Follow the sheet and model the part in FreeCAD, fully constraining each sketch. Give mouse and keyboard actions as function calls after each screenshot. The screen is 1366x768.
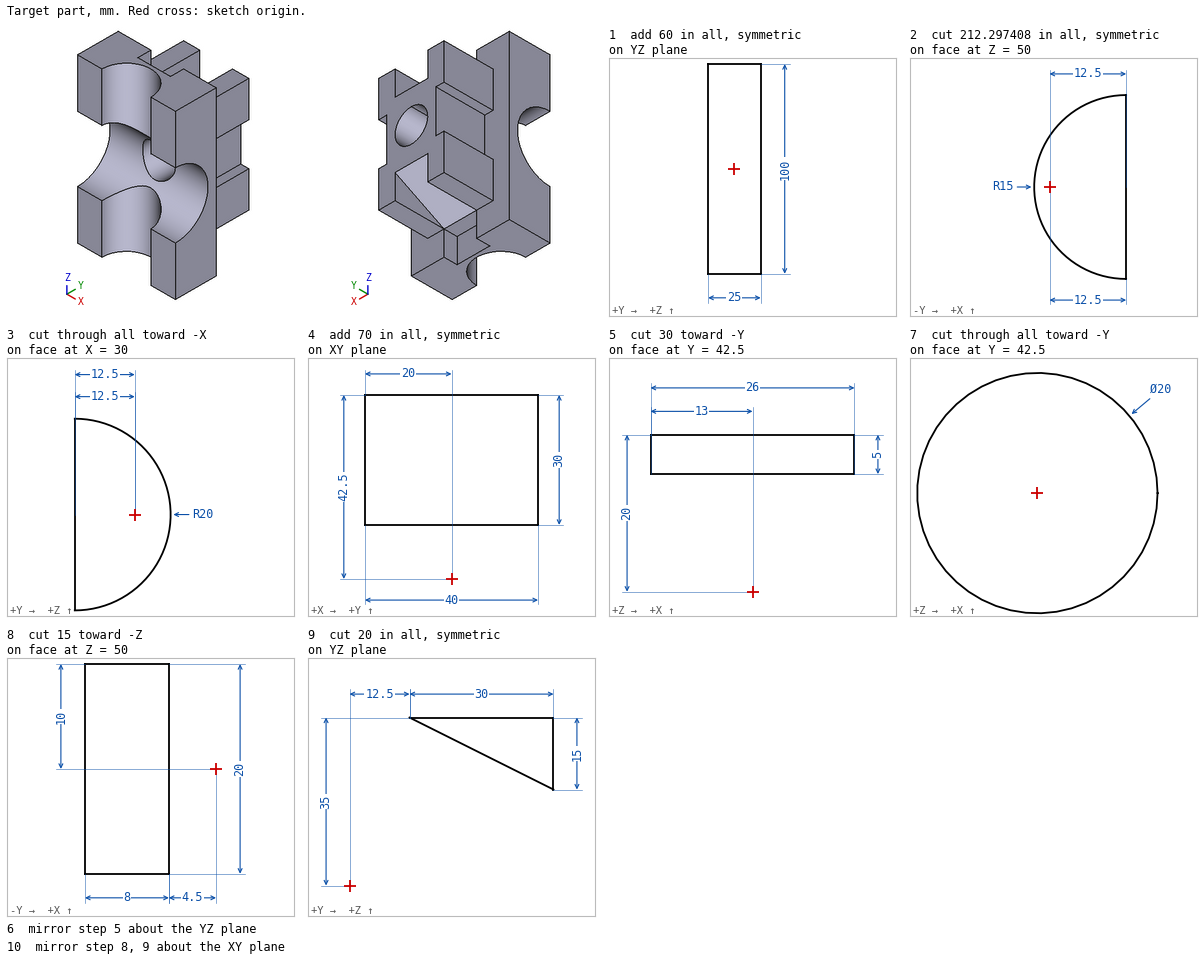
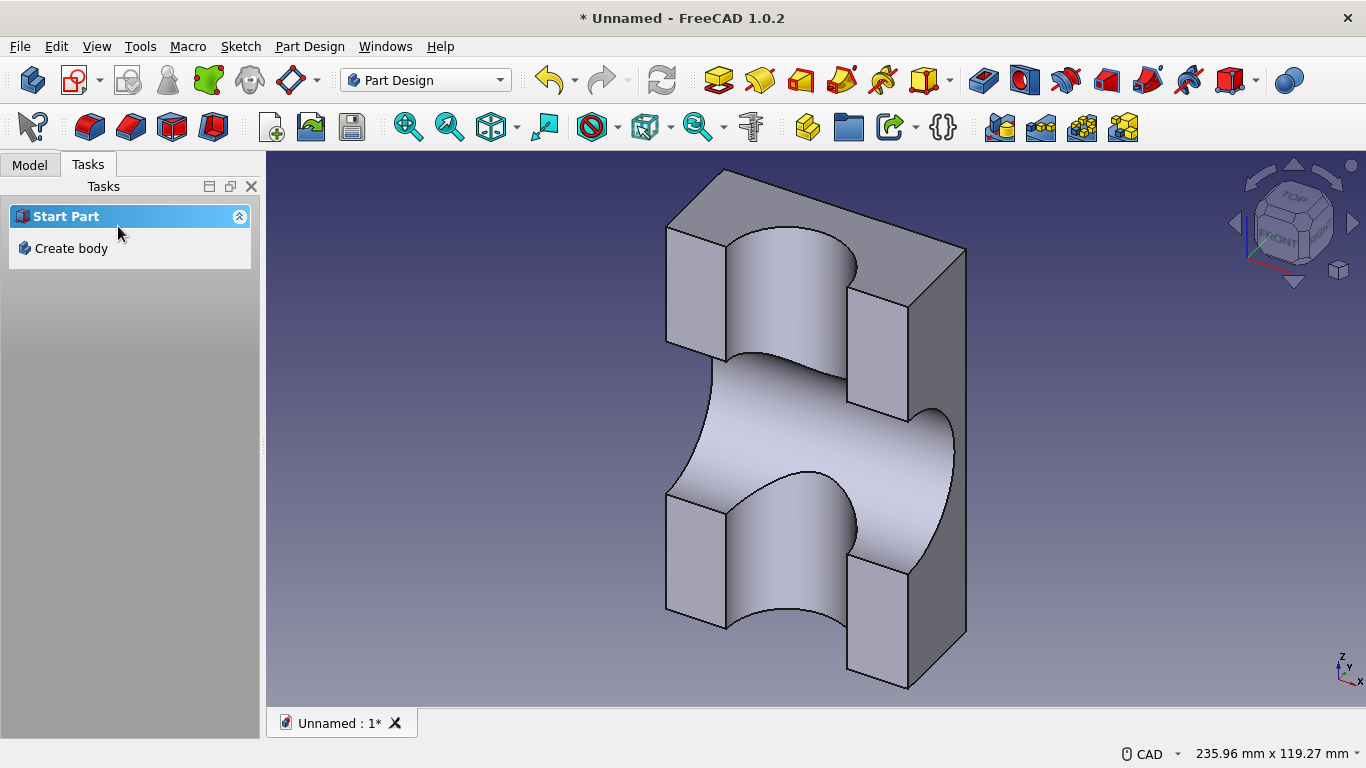
click(74, 80)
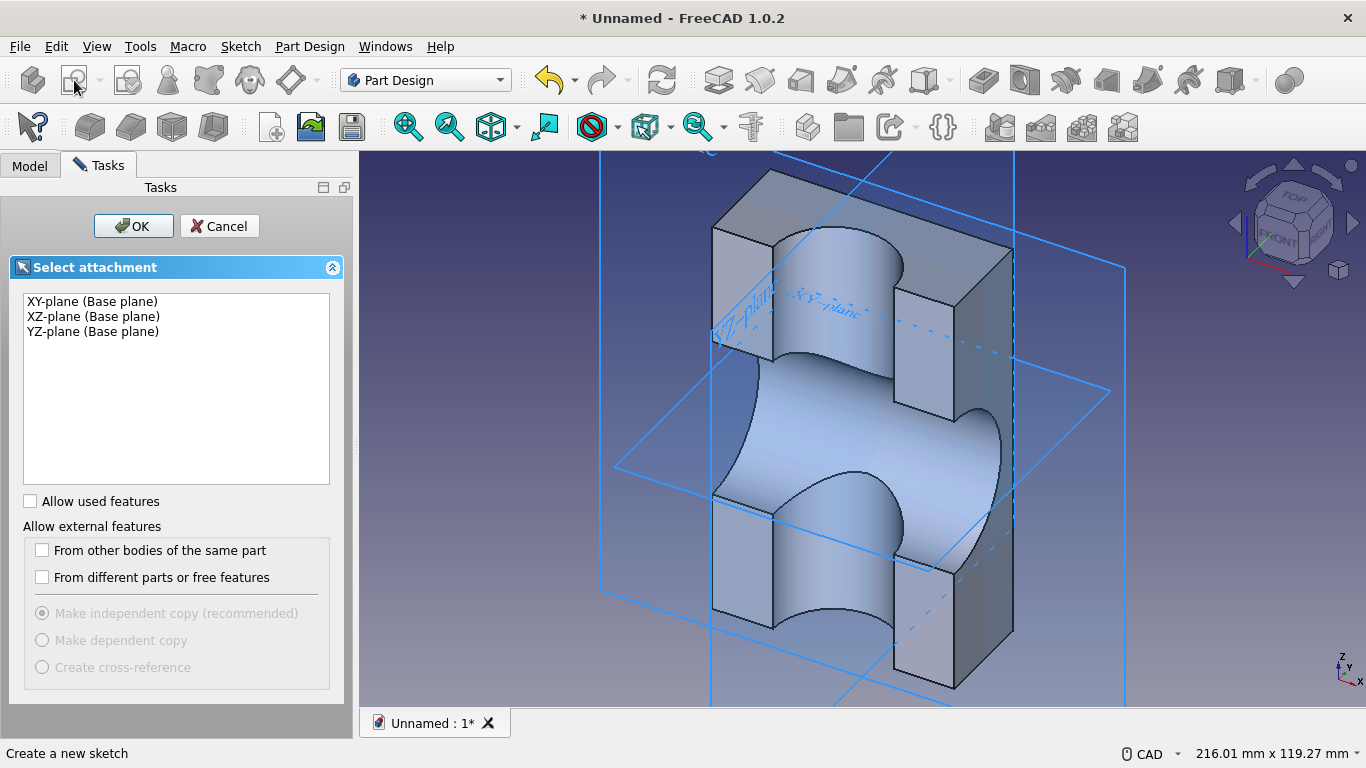
click(84, 302)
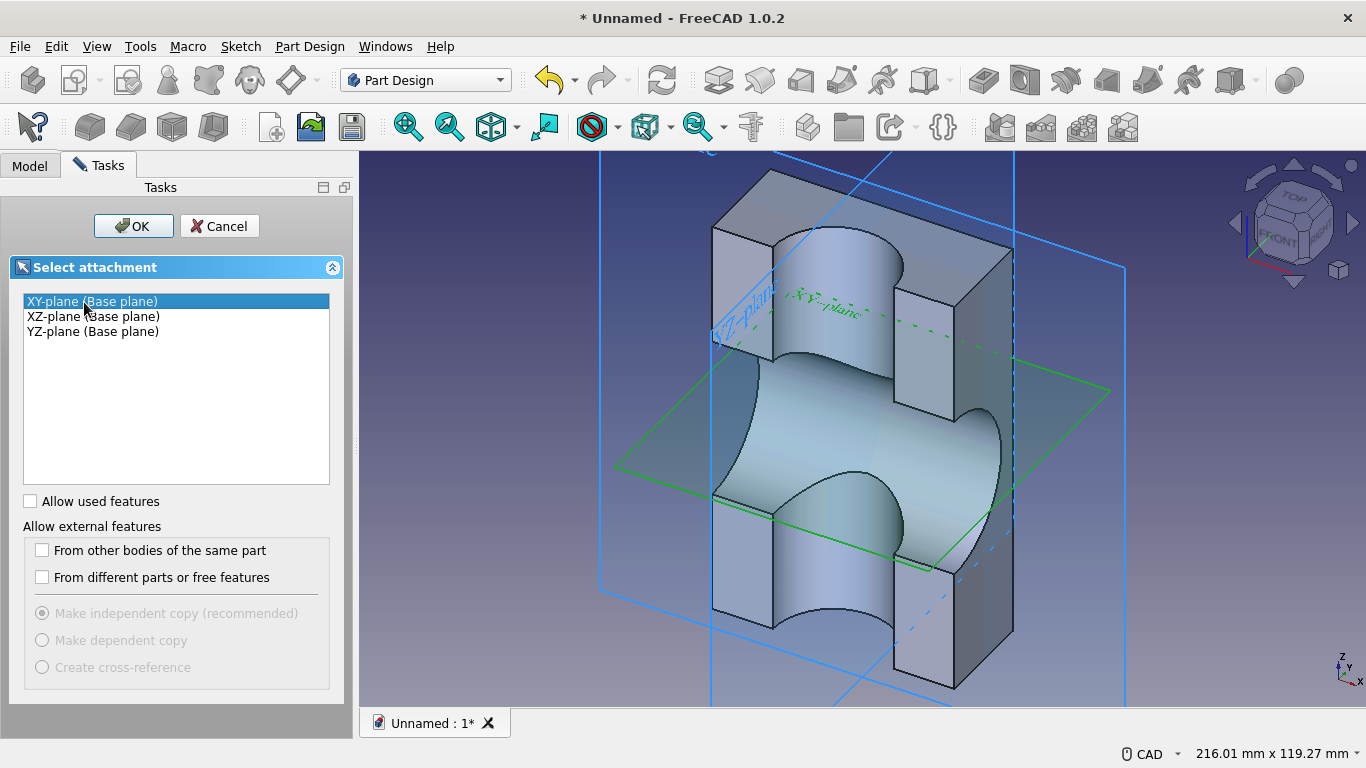
click(134, 226)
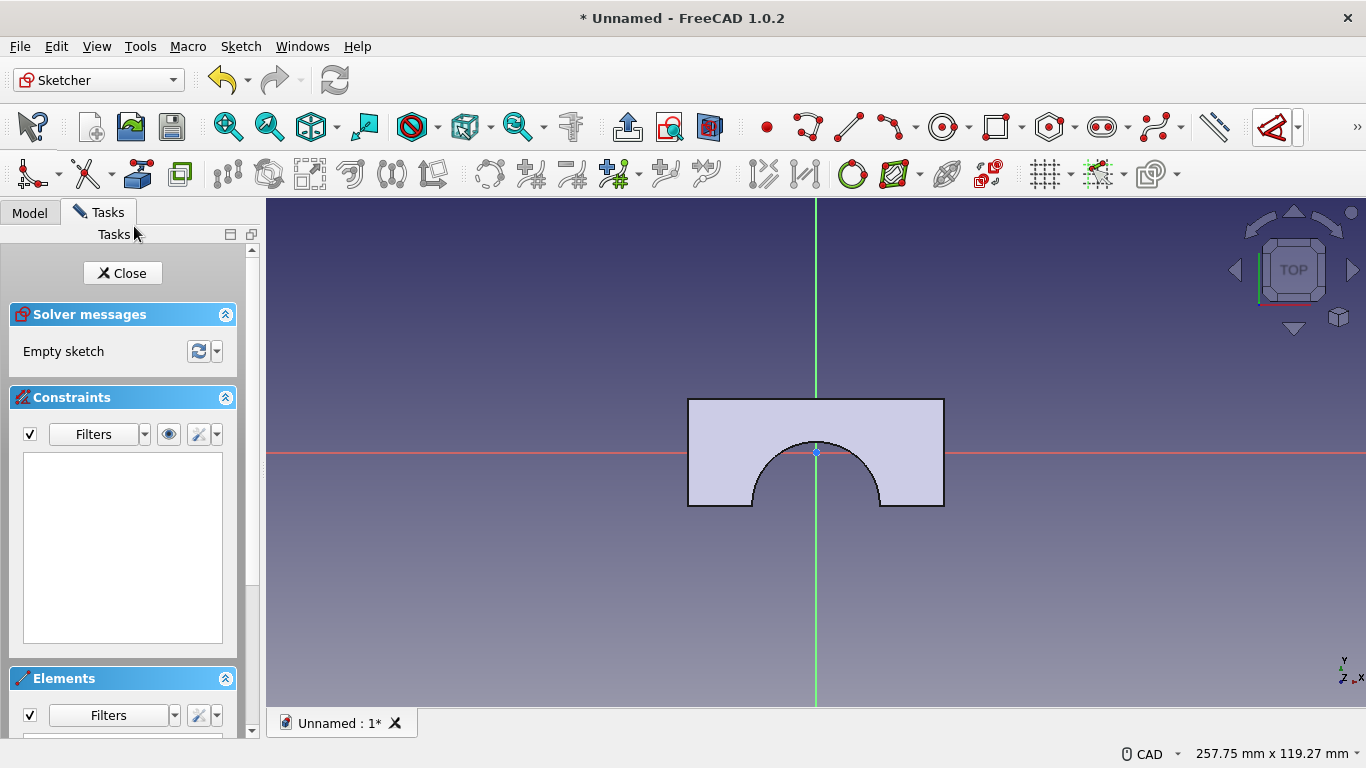
click(710, 128)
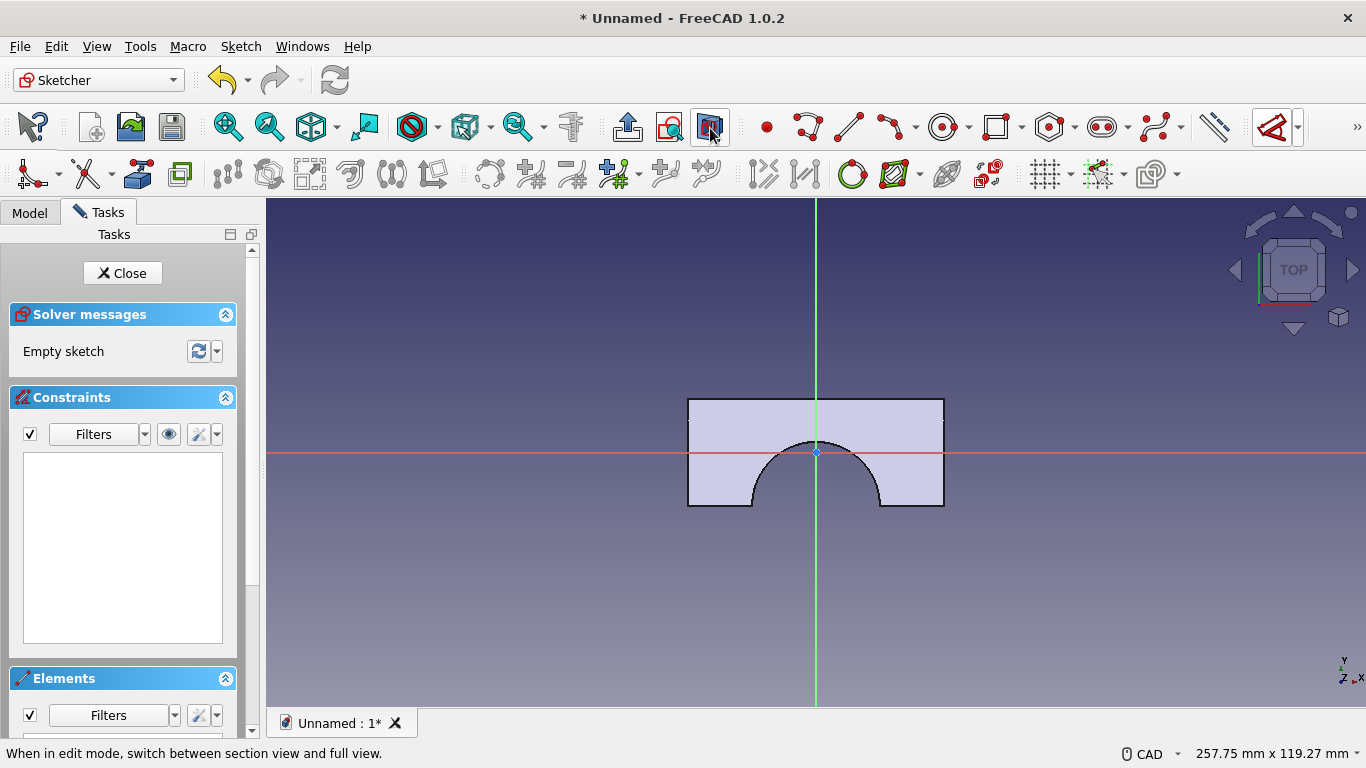
scroll(899, 252, up, 3)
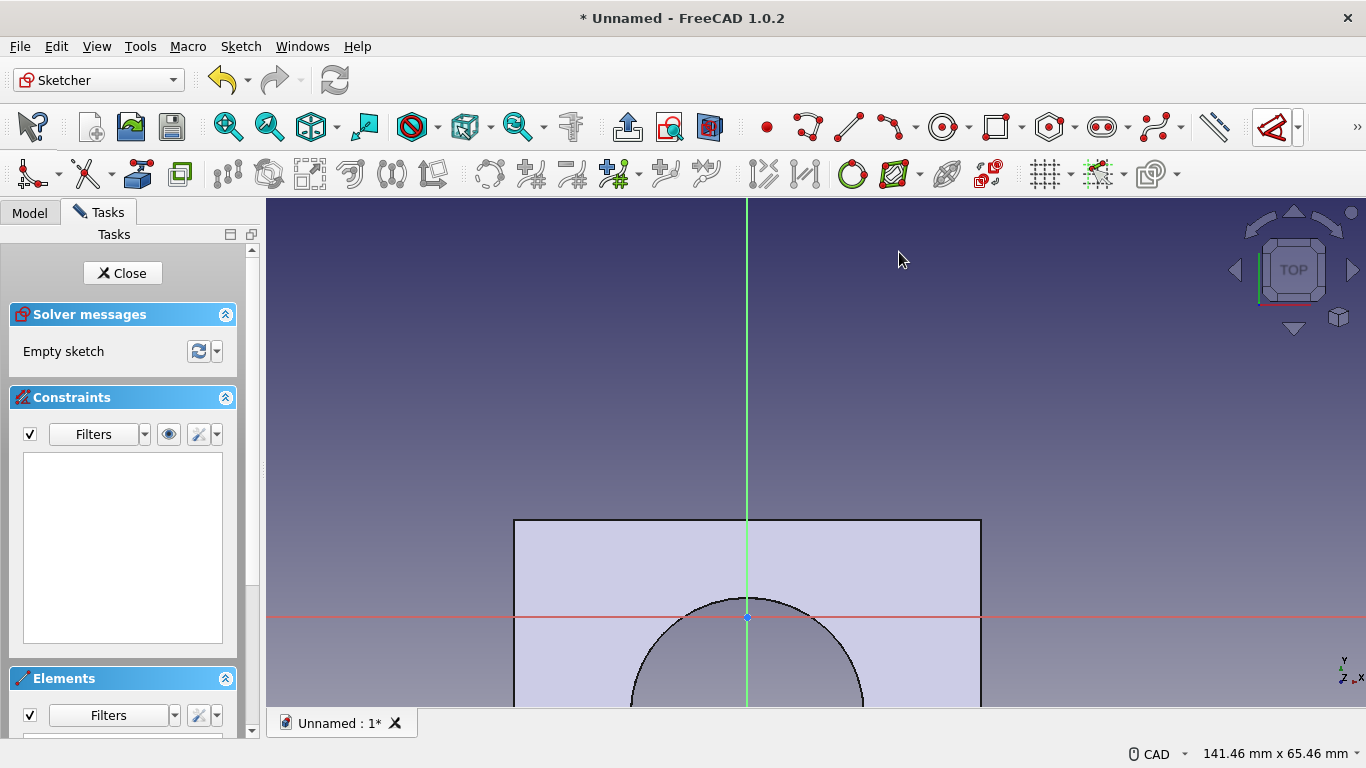
click(996, 128)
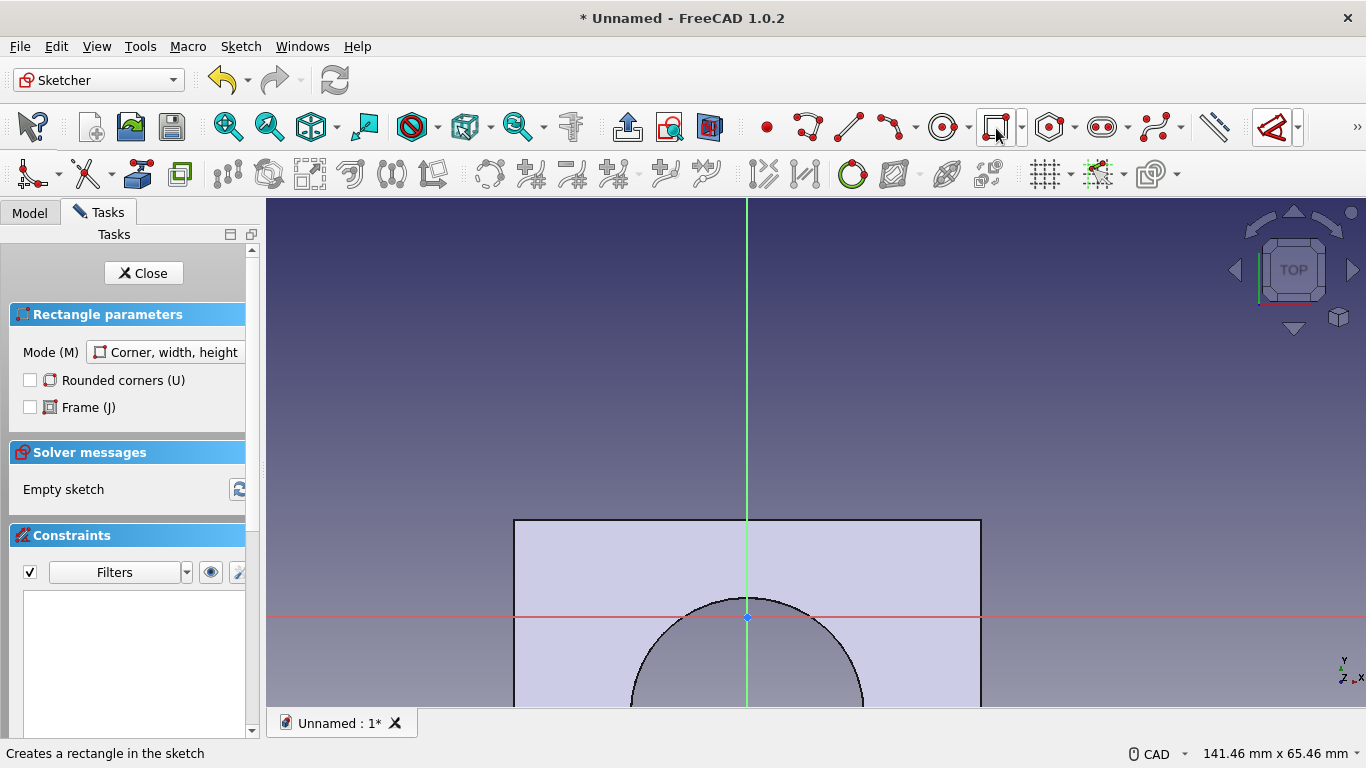
click(592, 287)
move(903, 520)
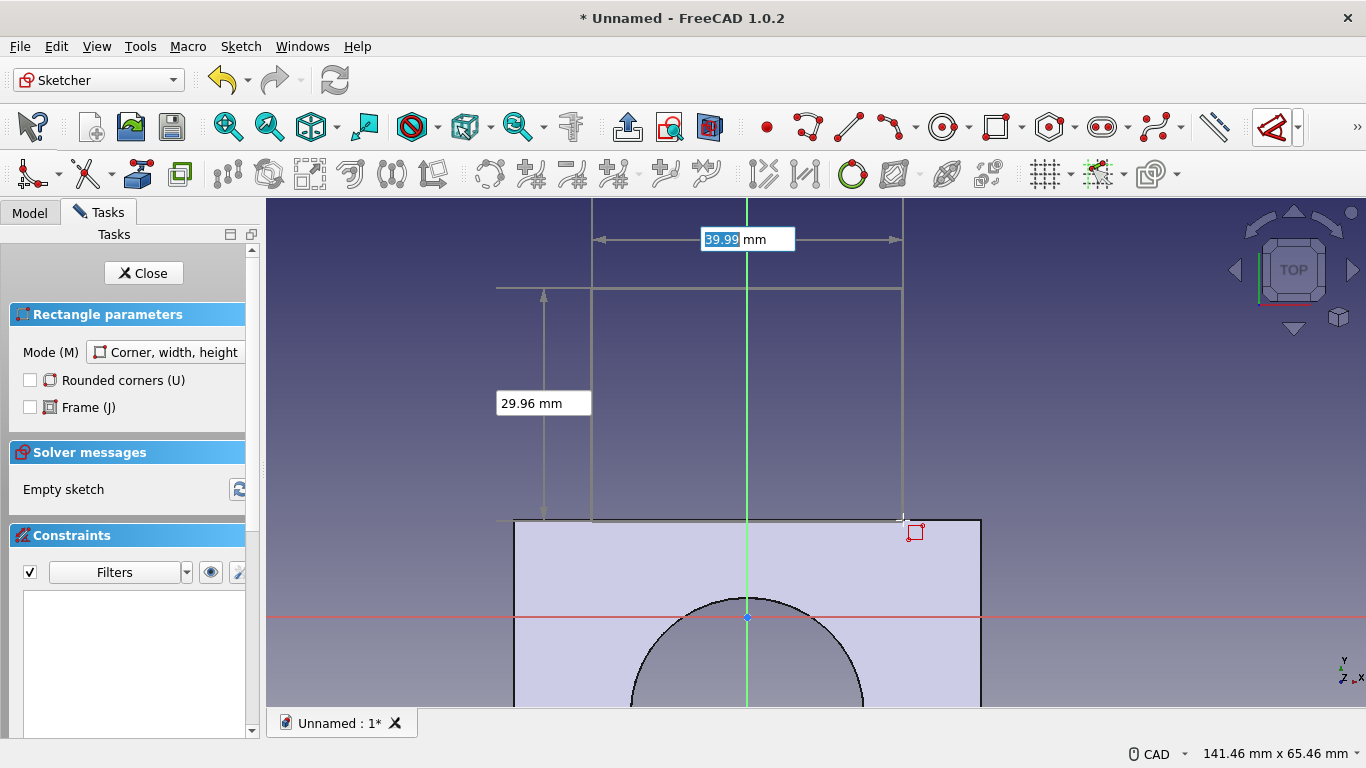
text(40)
key(Tab)
text(30)
key(Return)
key(Escape)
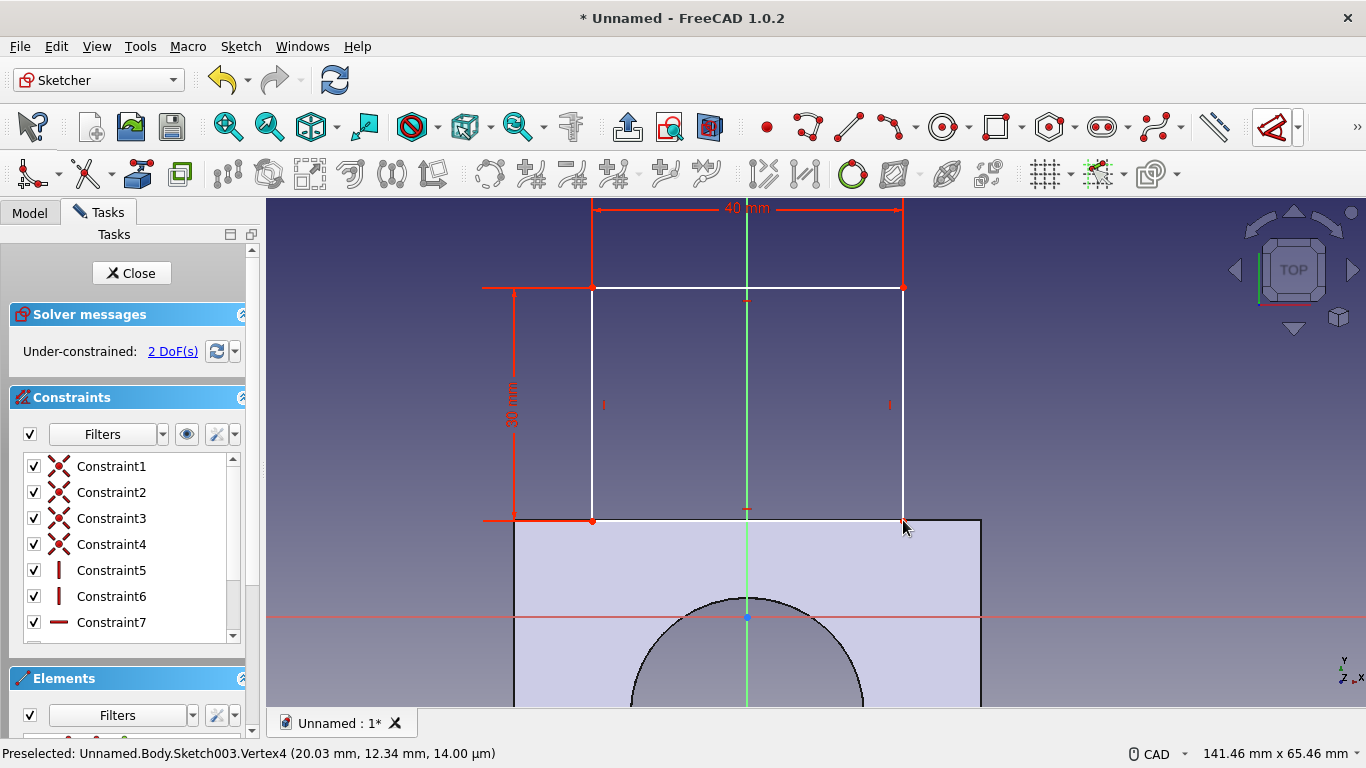
click(592, 288)